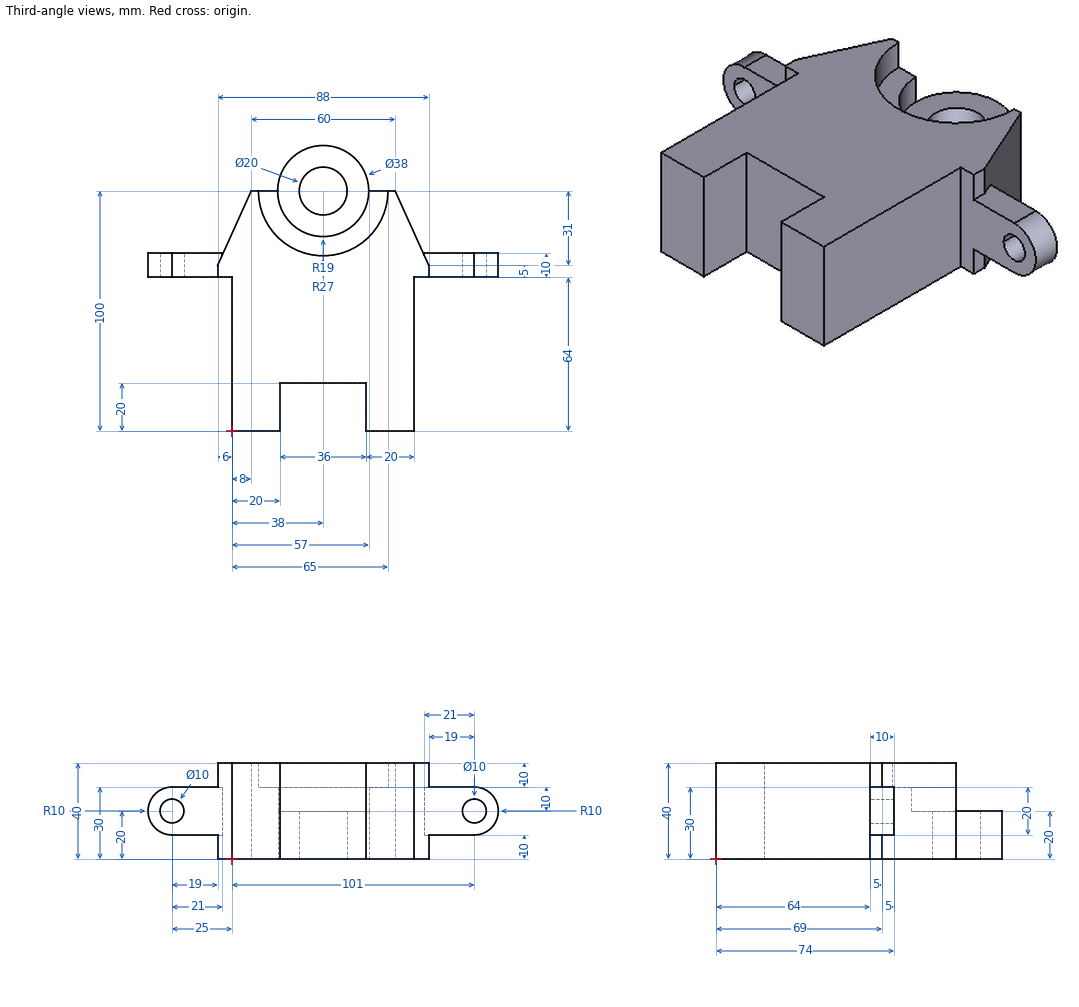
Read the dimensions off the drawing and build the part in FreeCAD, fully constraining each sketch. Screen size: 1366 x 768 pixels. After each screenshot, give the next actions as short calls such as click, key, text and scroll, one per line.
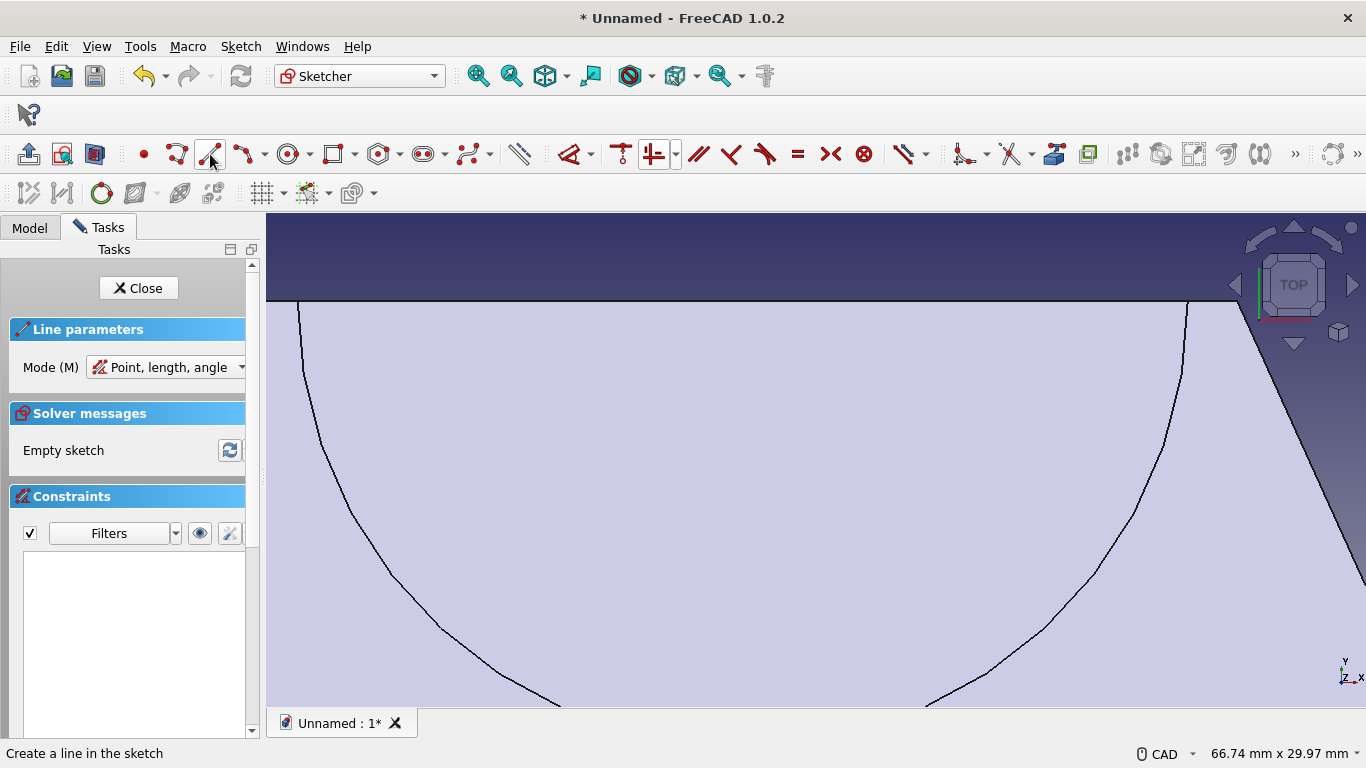
click(1056, 301)
click(430, 301)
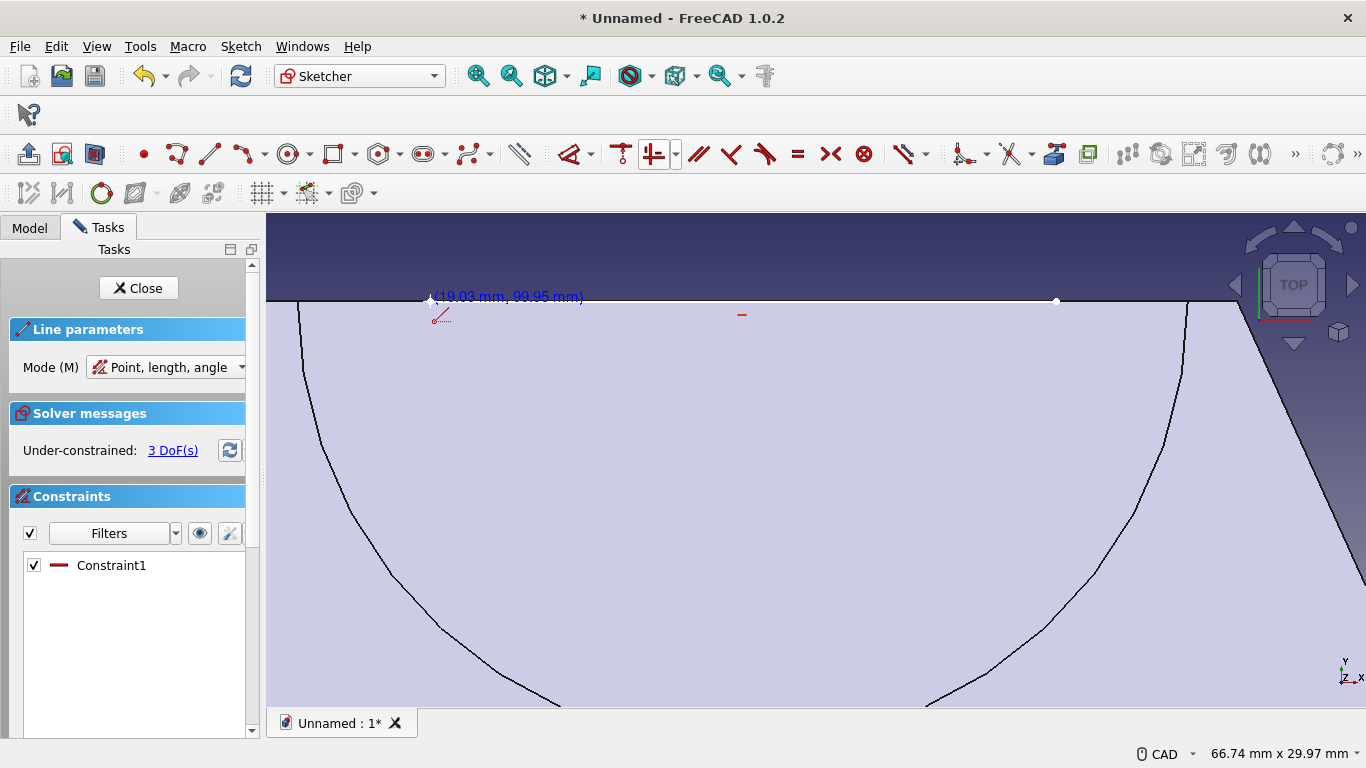
click(242, 154)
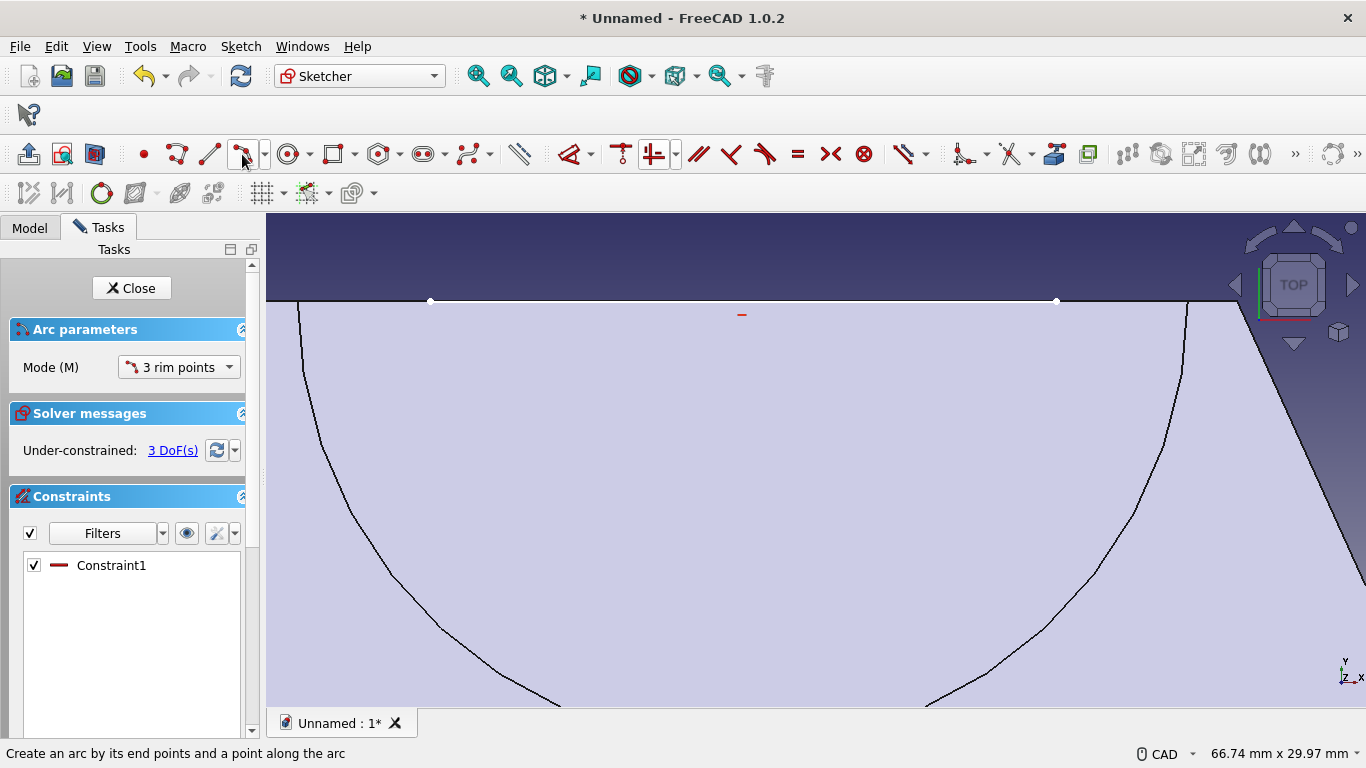
click(430, 302)
click(1056, 302)
click(743, 614)
key(Escape)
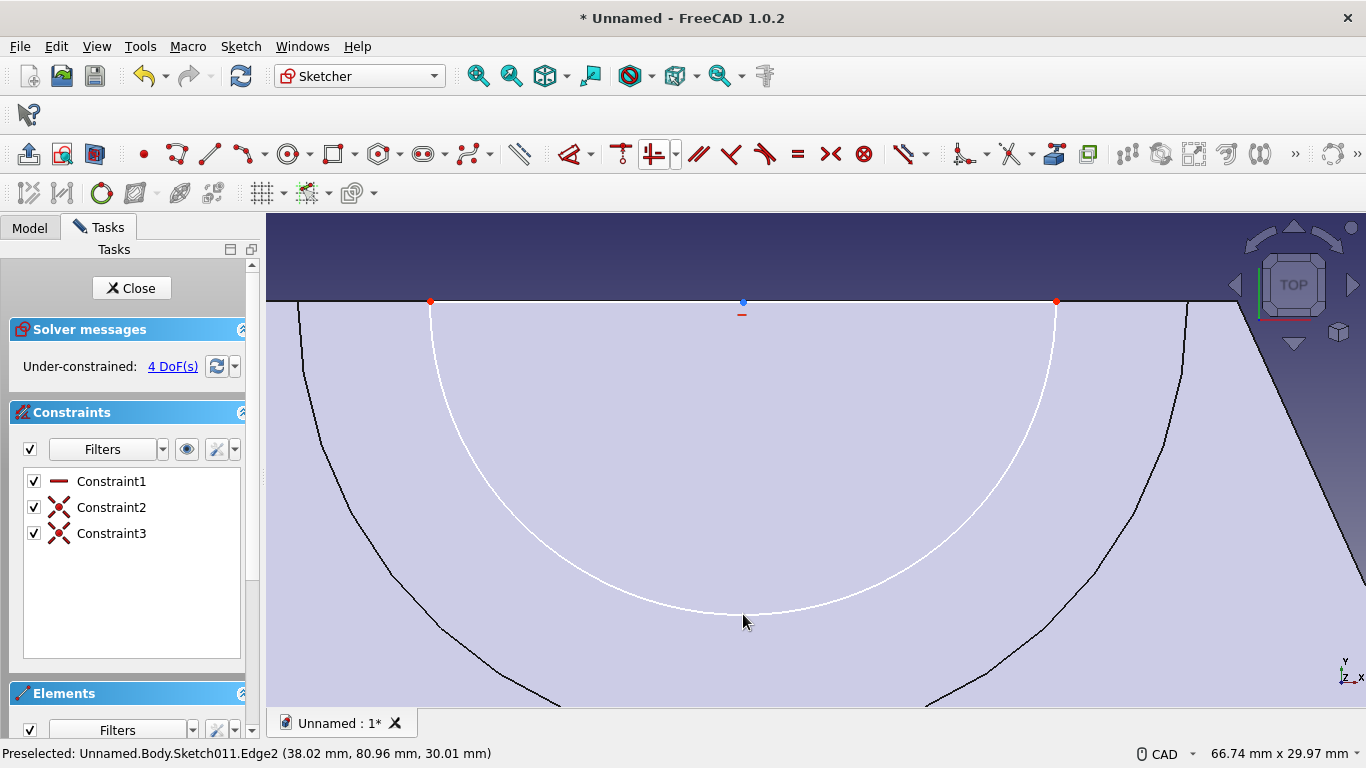
click(568, 154)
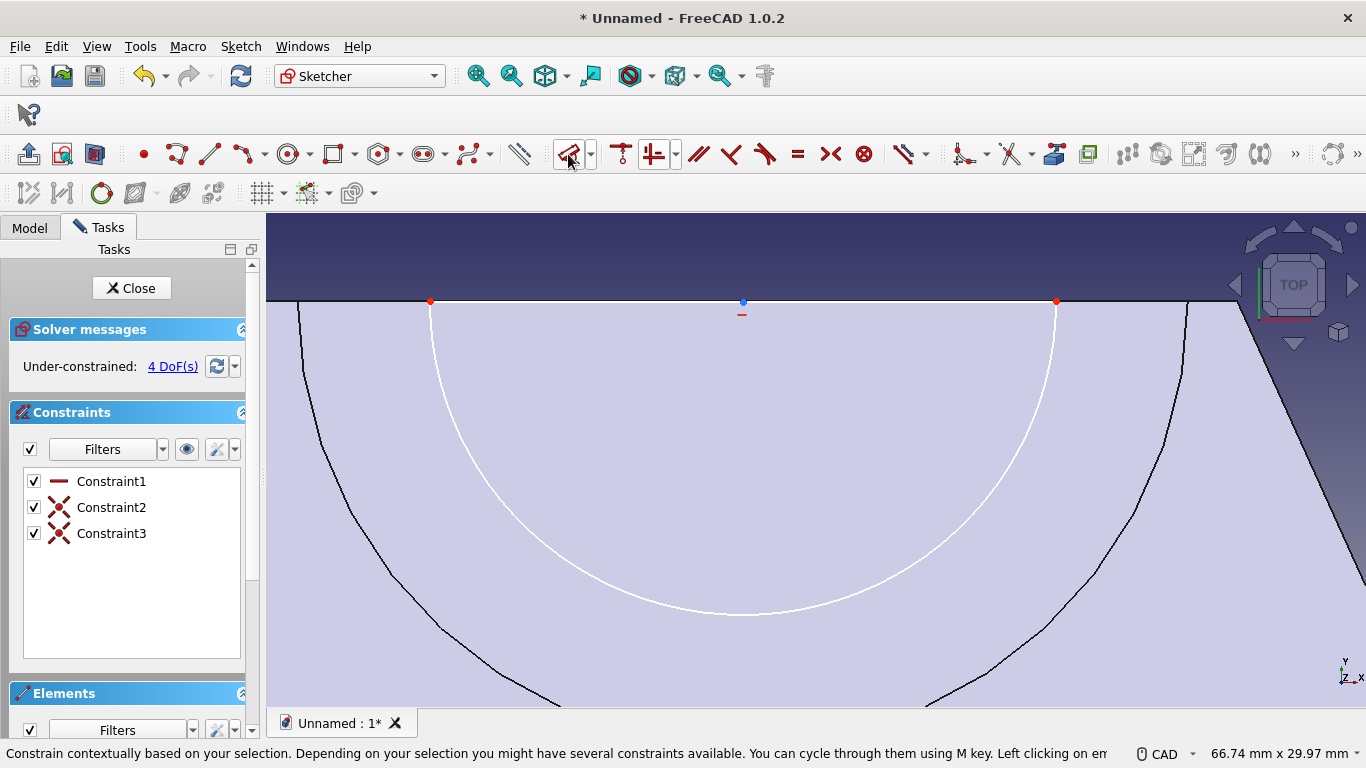
click(559, 555)
click(540, 581)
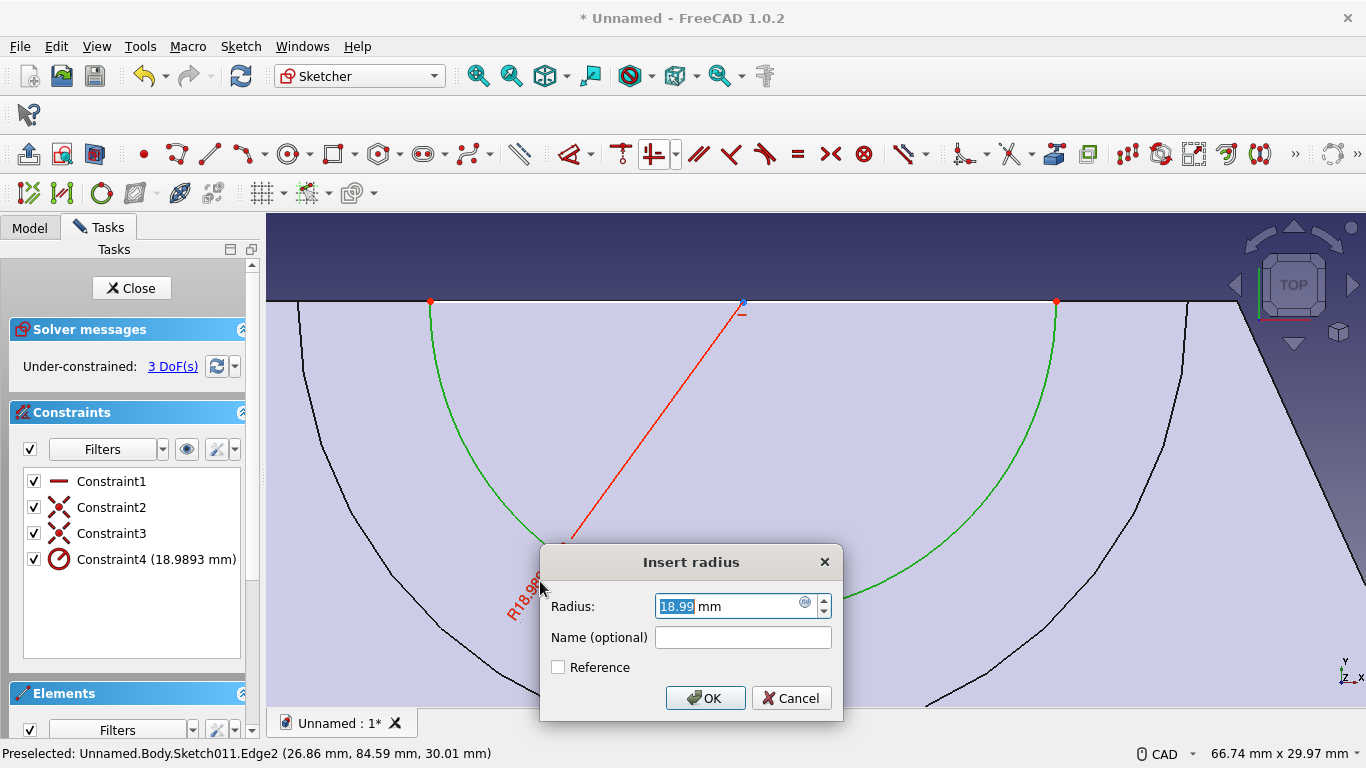
text(19)
key(Return)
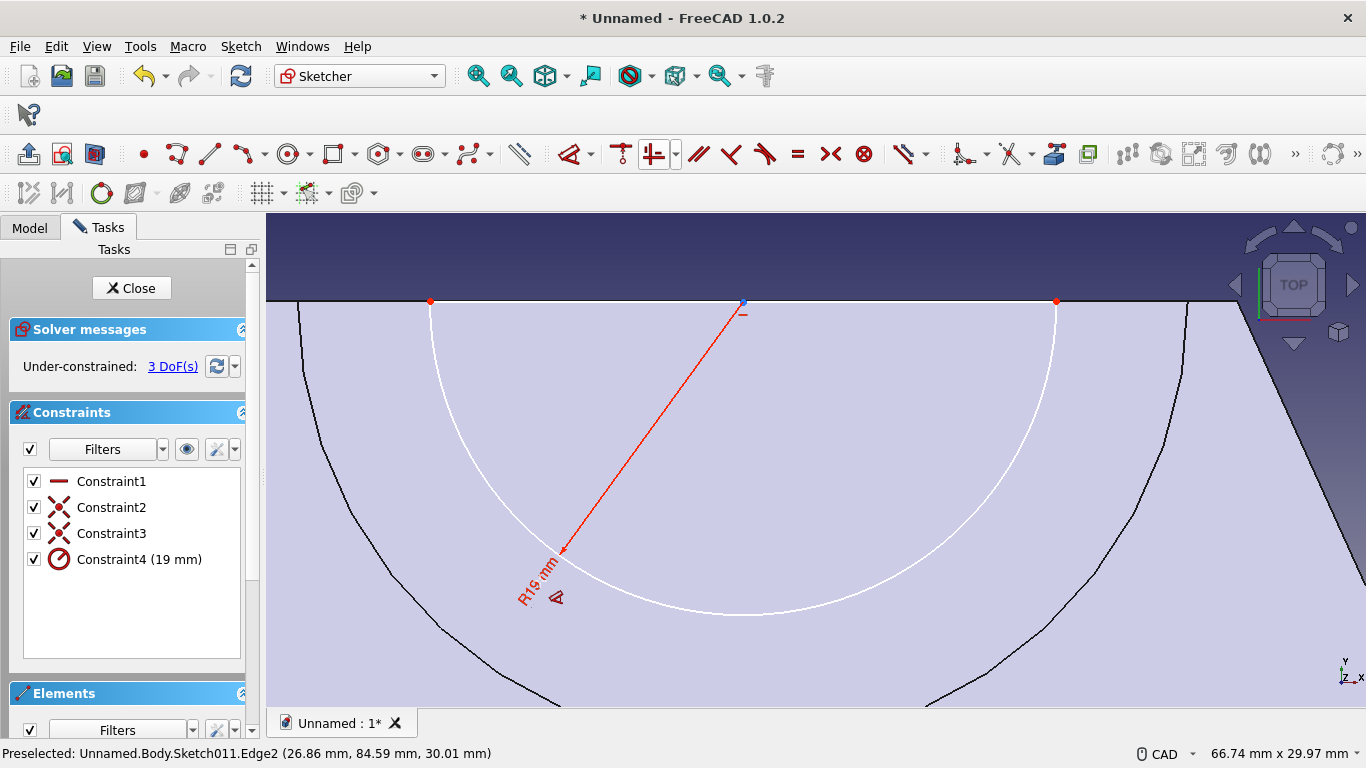
click(1056, 302)
click(675, 268)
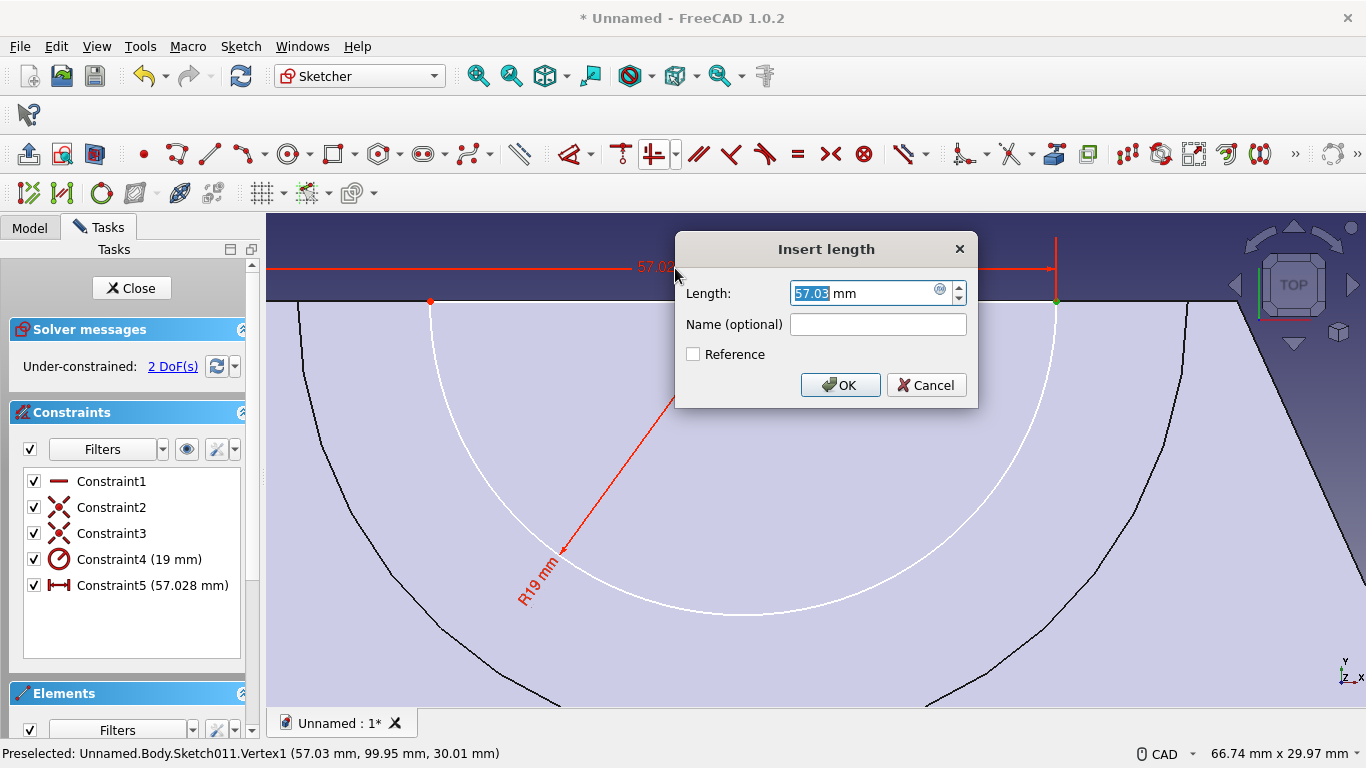
text(57)
key(Return)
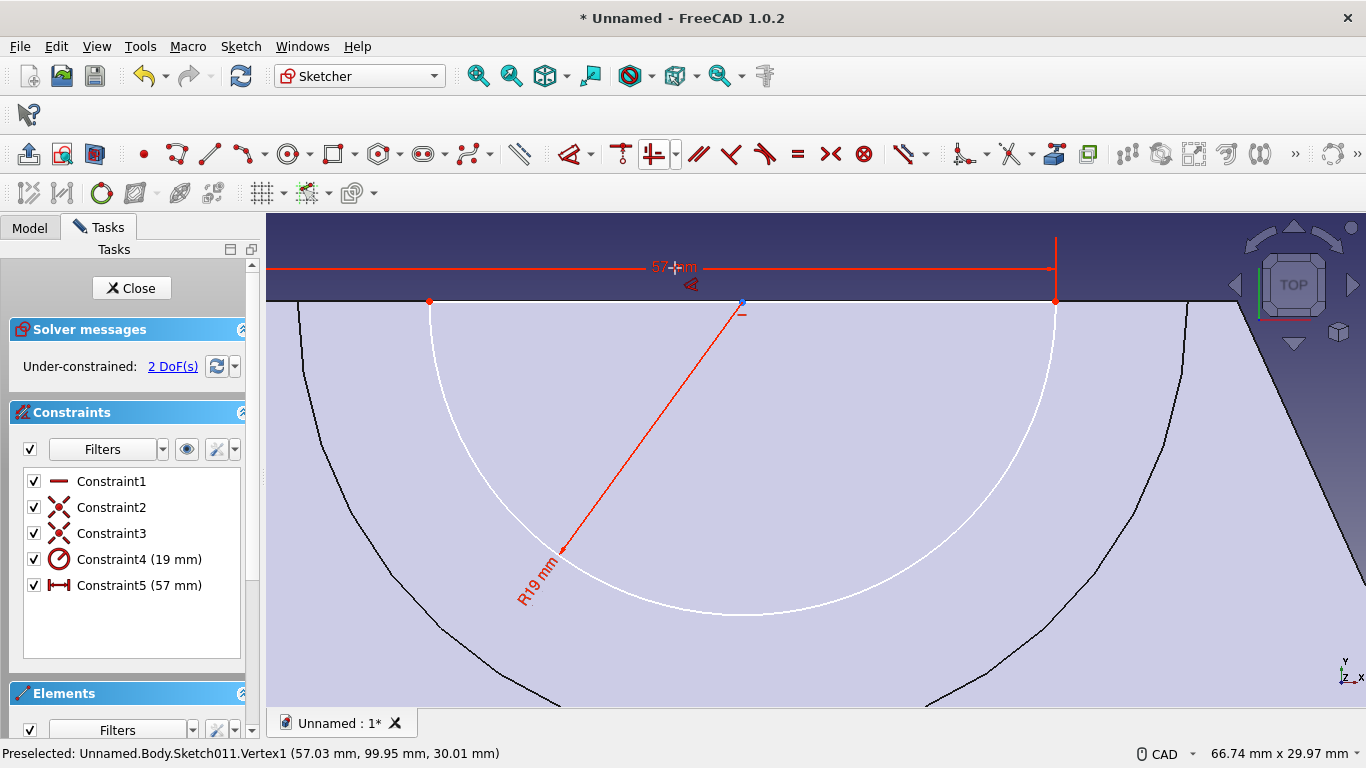
click(1056, 302)
click(1090, 490)